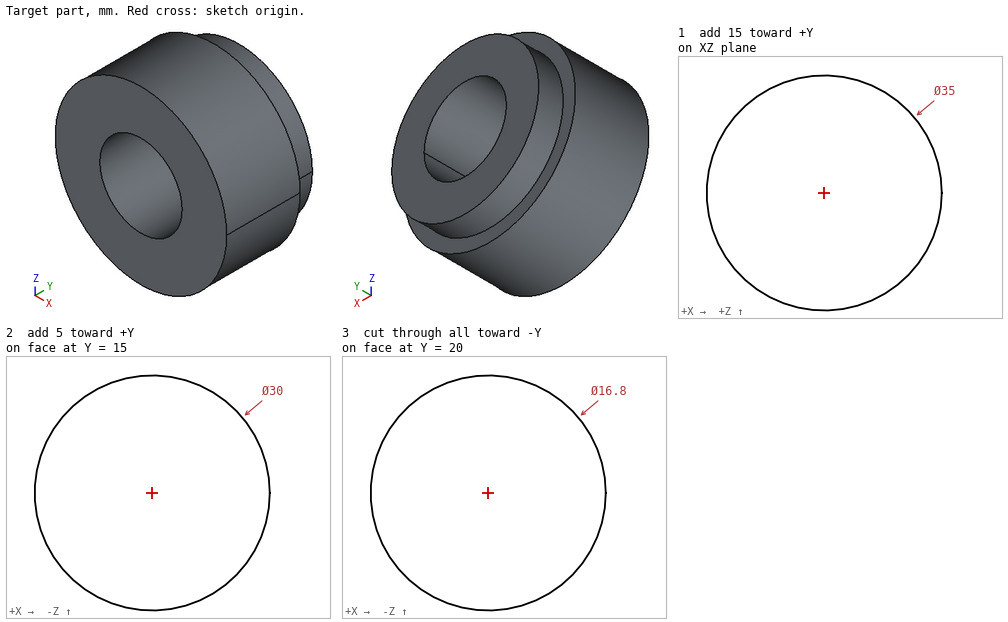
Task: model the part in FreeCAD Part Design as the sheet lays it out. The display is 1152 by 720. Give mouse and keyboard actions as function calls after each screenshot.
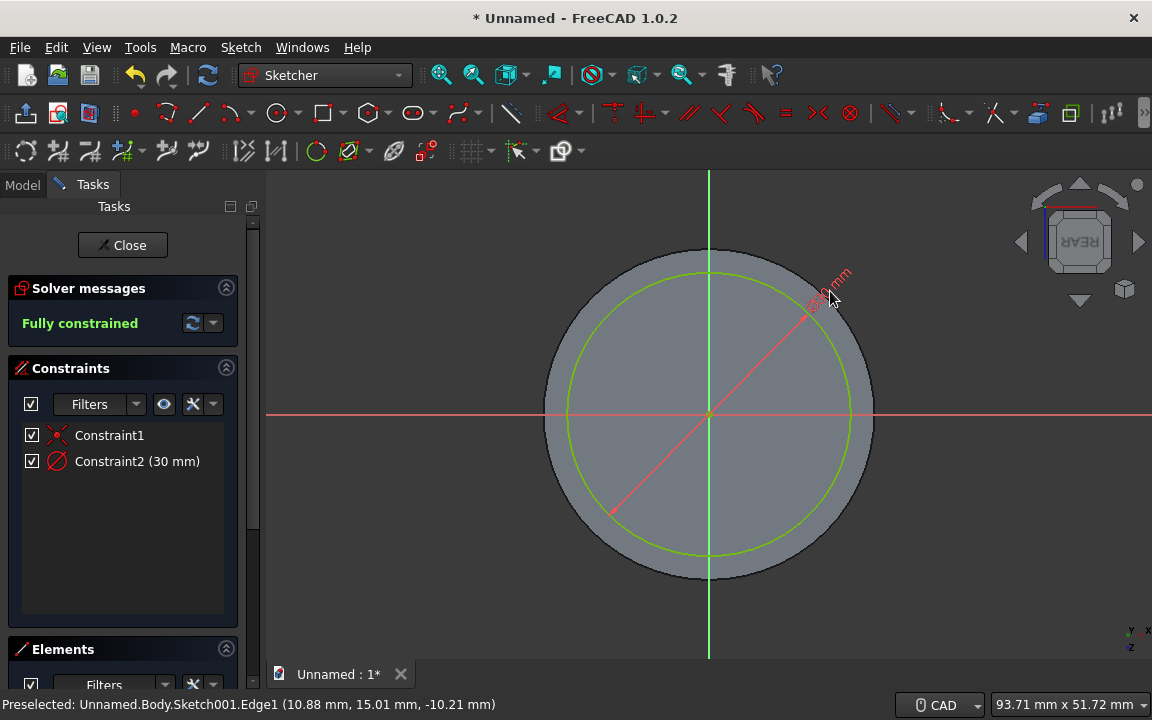
click(123, 245)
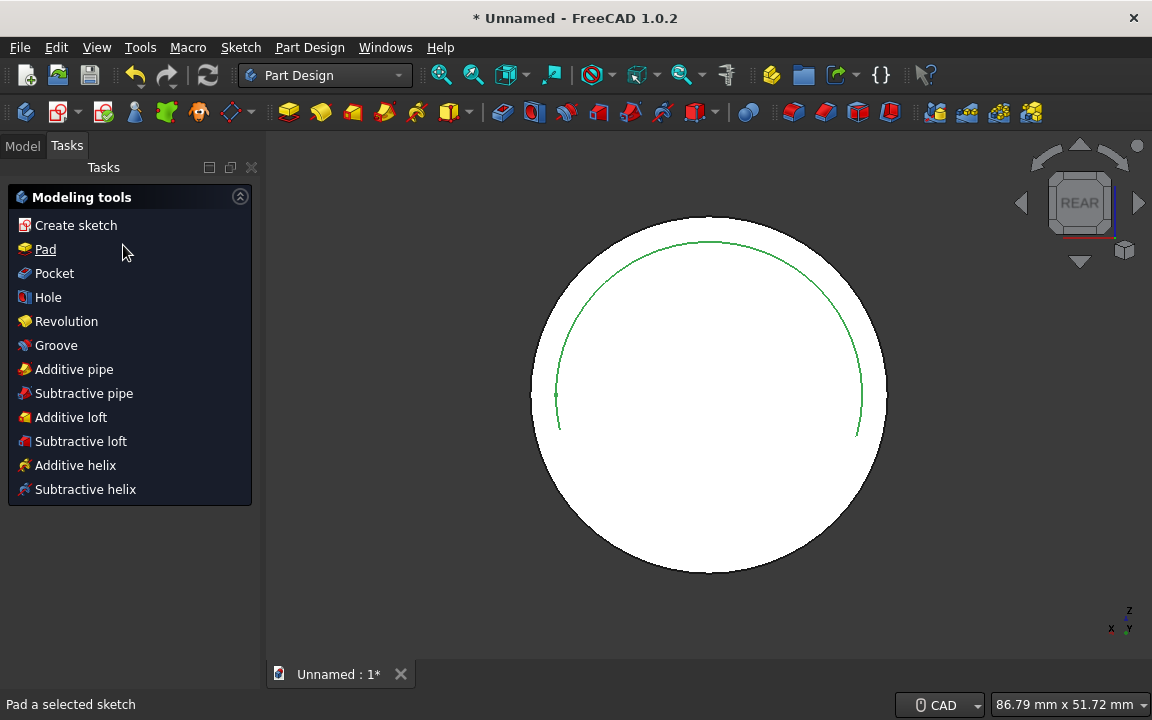
click(290, 112)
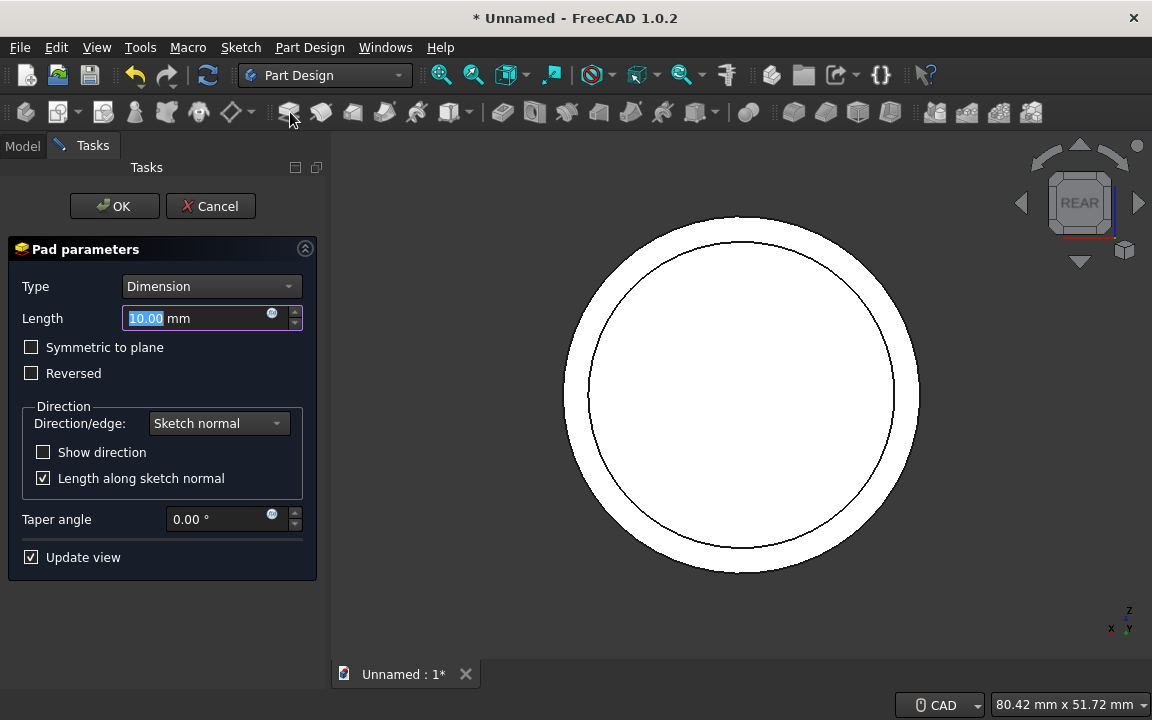
text(5)
key(Tab)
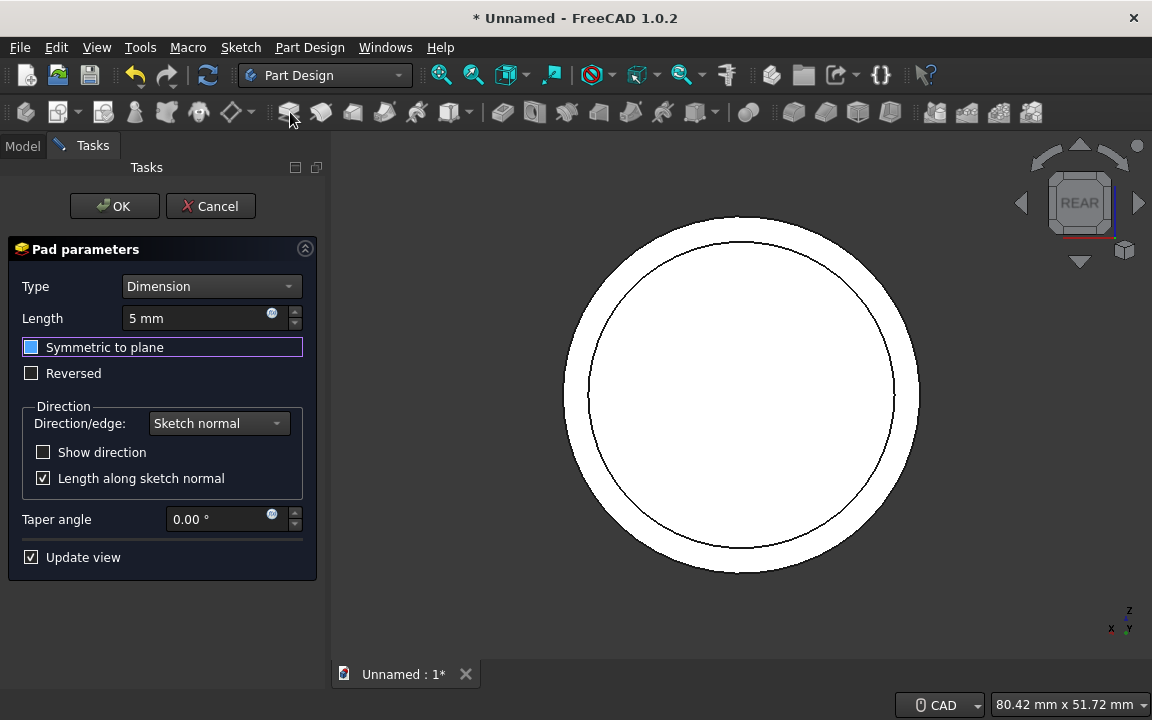
click(115, 206)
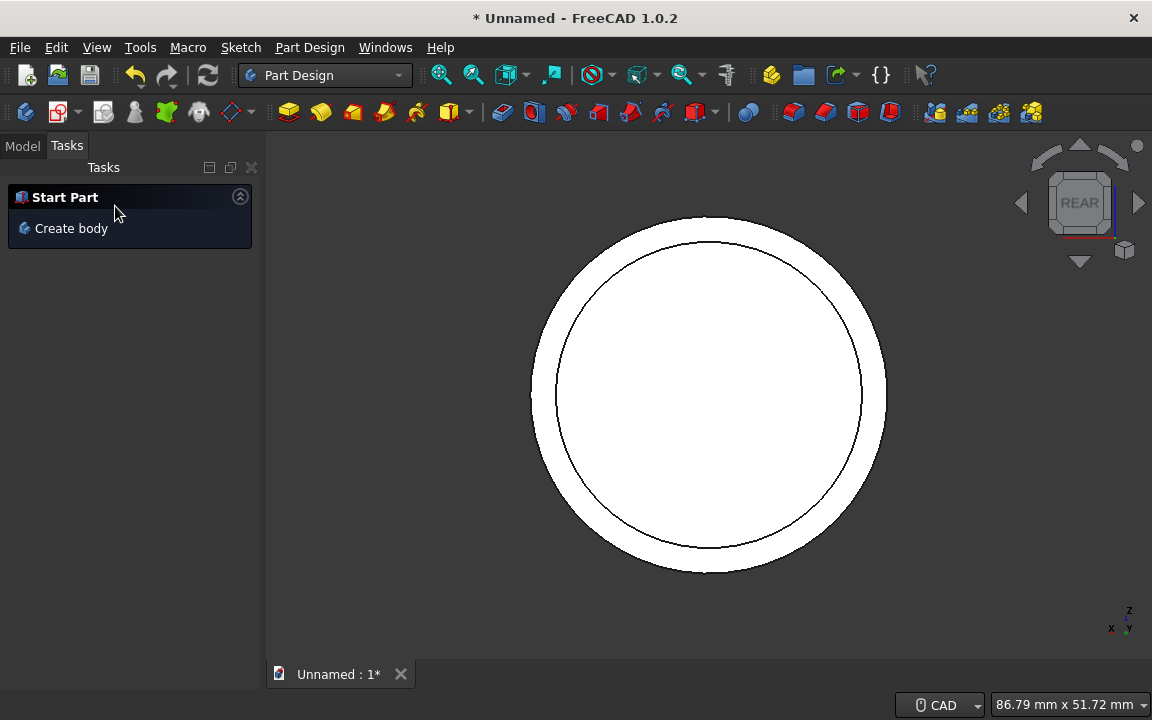
click(709, 394)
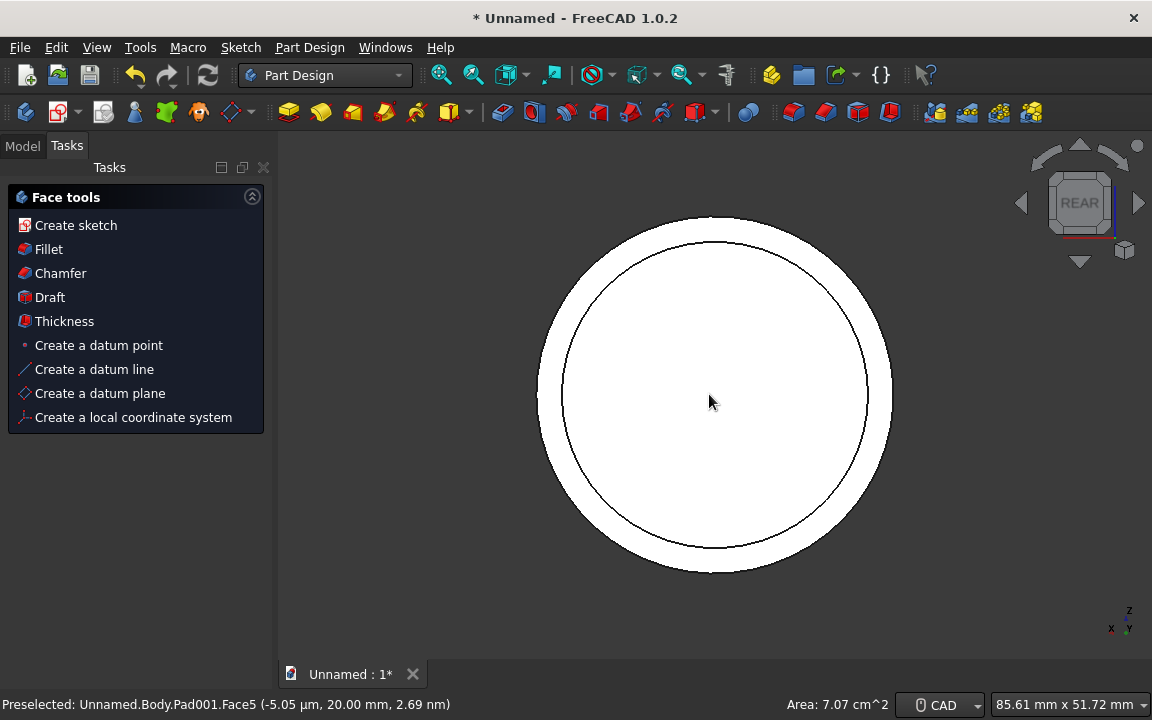
click(58, 112)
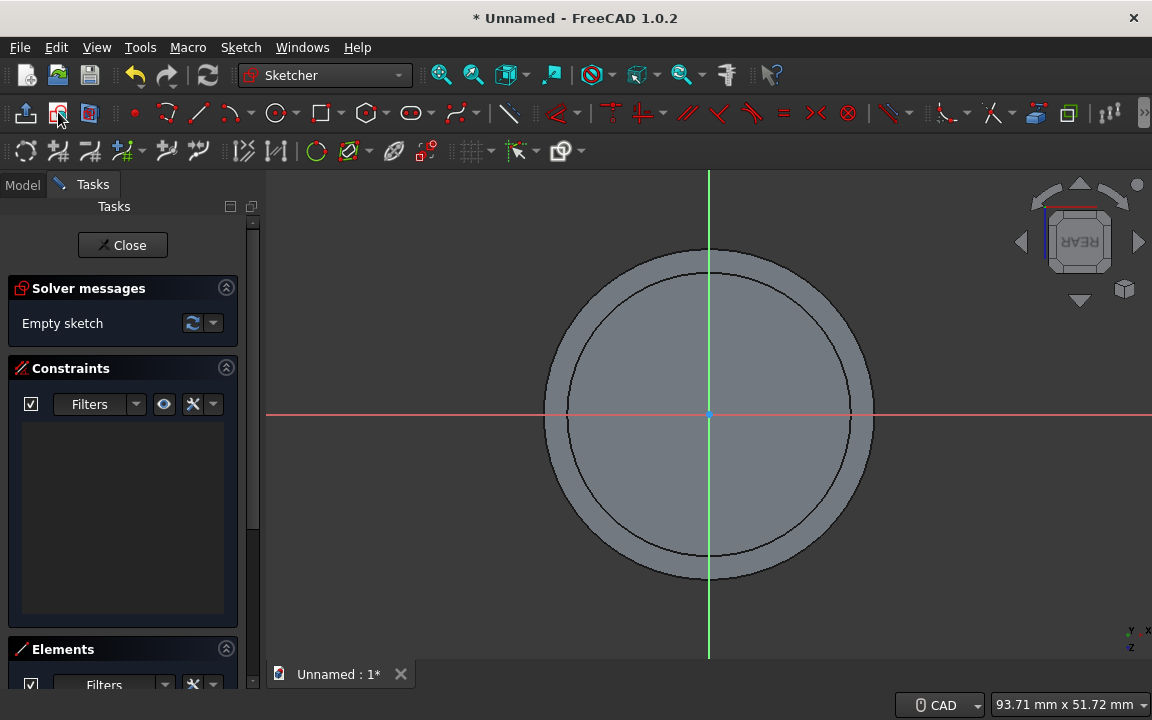
scroll(792, 414, up, 3)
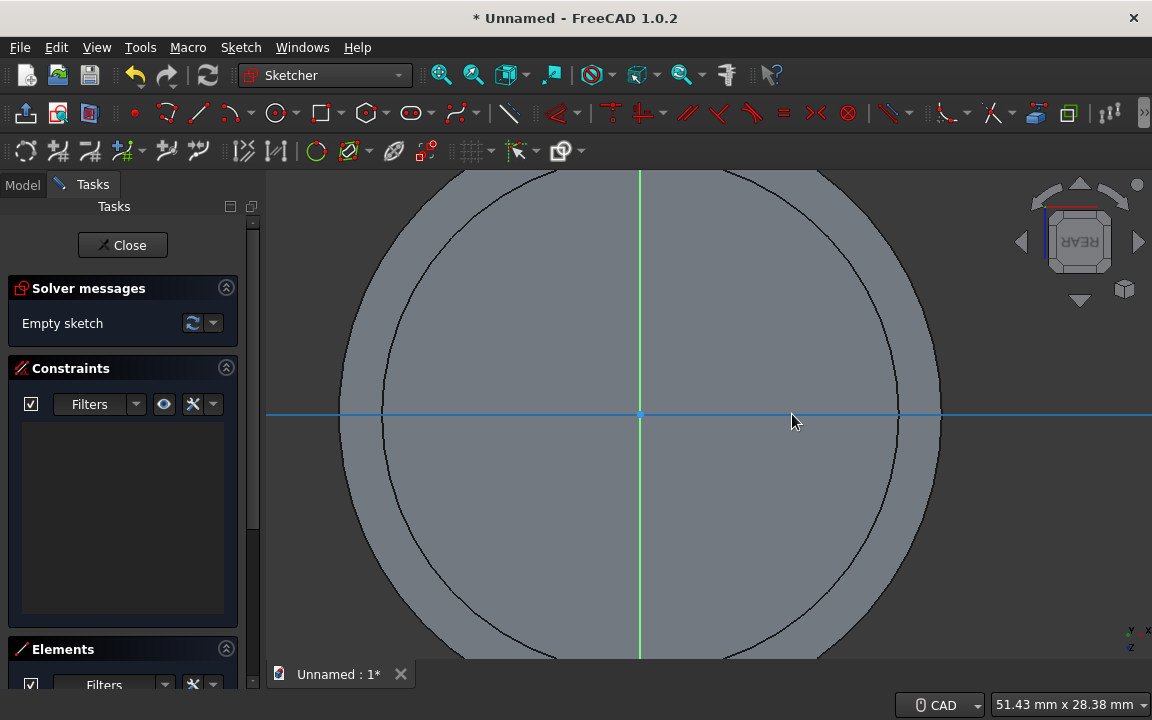
click(276, 114)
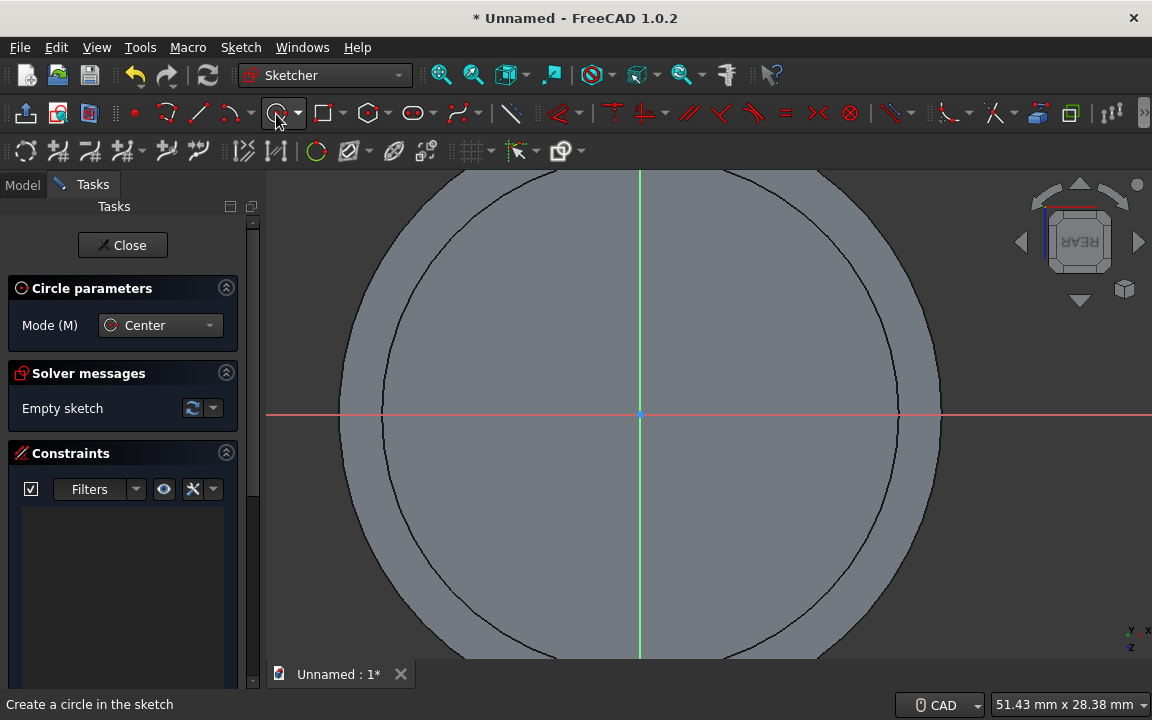
click(640, 414)
click(743, 312)
key(Escape)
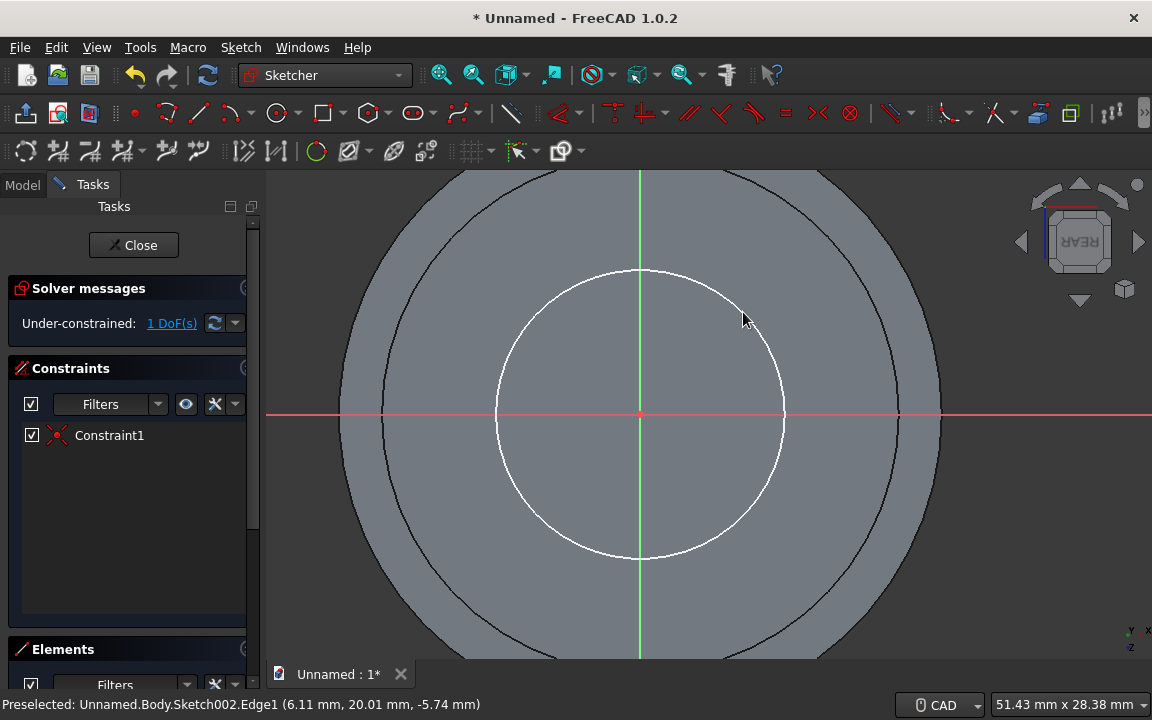
click(558, 114)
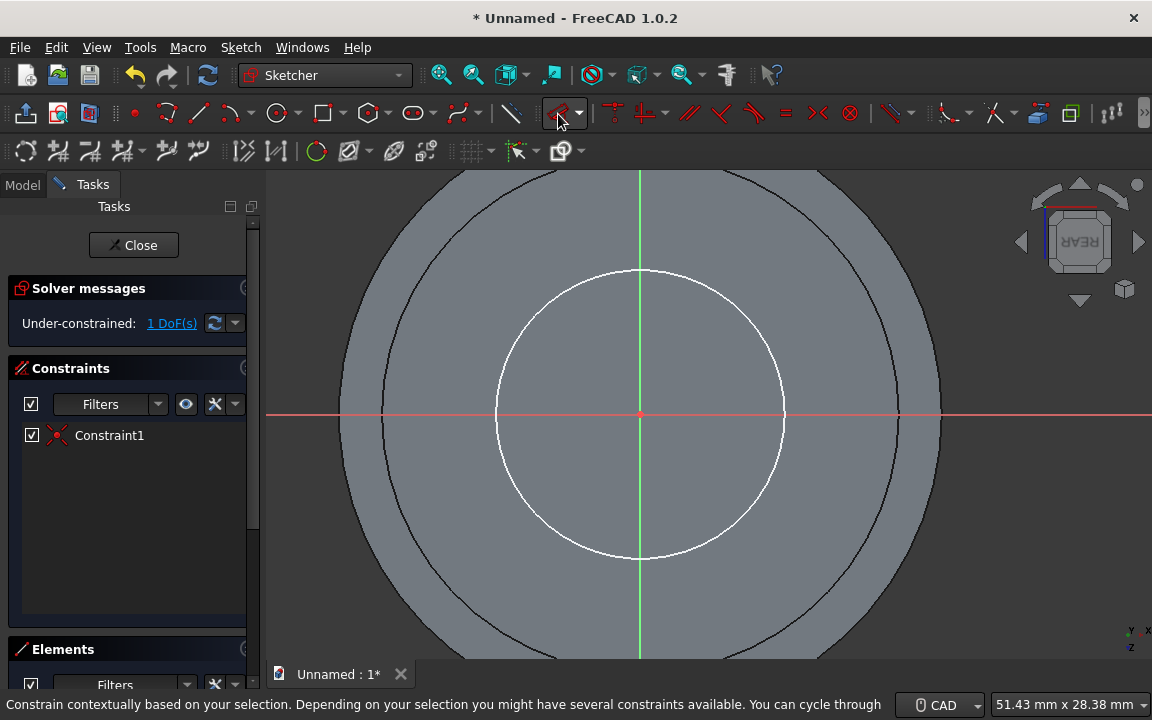
click(742, 312)
click(765, 289)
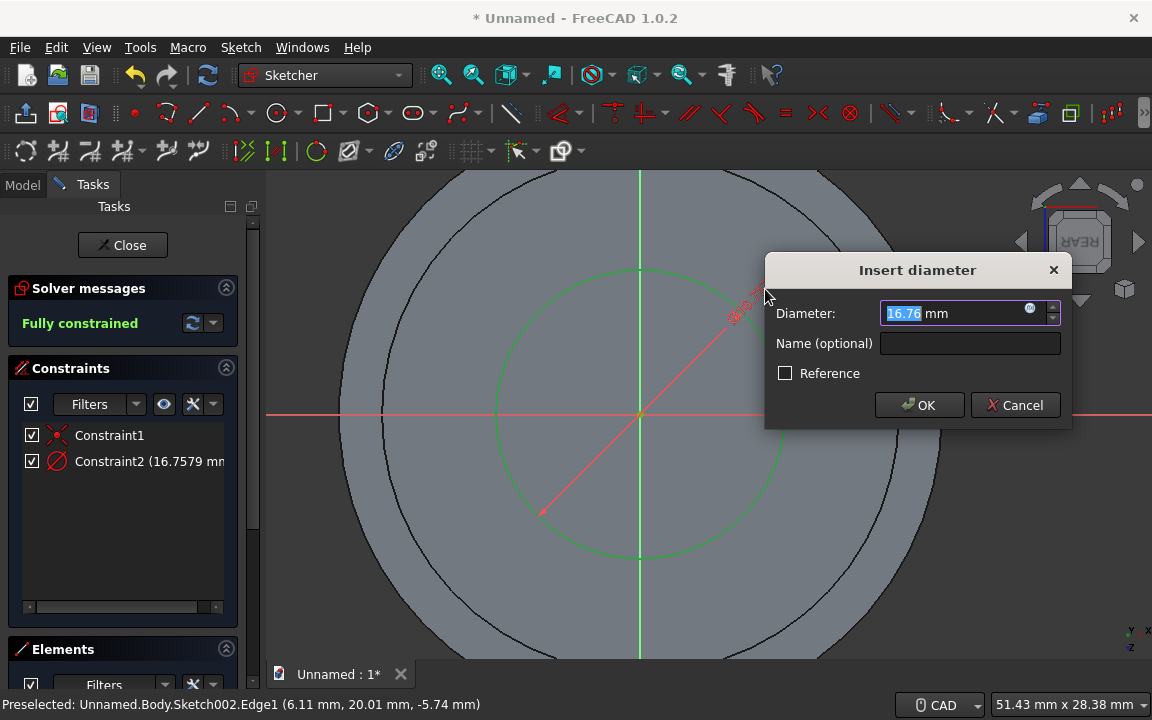
text(16.8)
key(Return)
key(Escape)